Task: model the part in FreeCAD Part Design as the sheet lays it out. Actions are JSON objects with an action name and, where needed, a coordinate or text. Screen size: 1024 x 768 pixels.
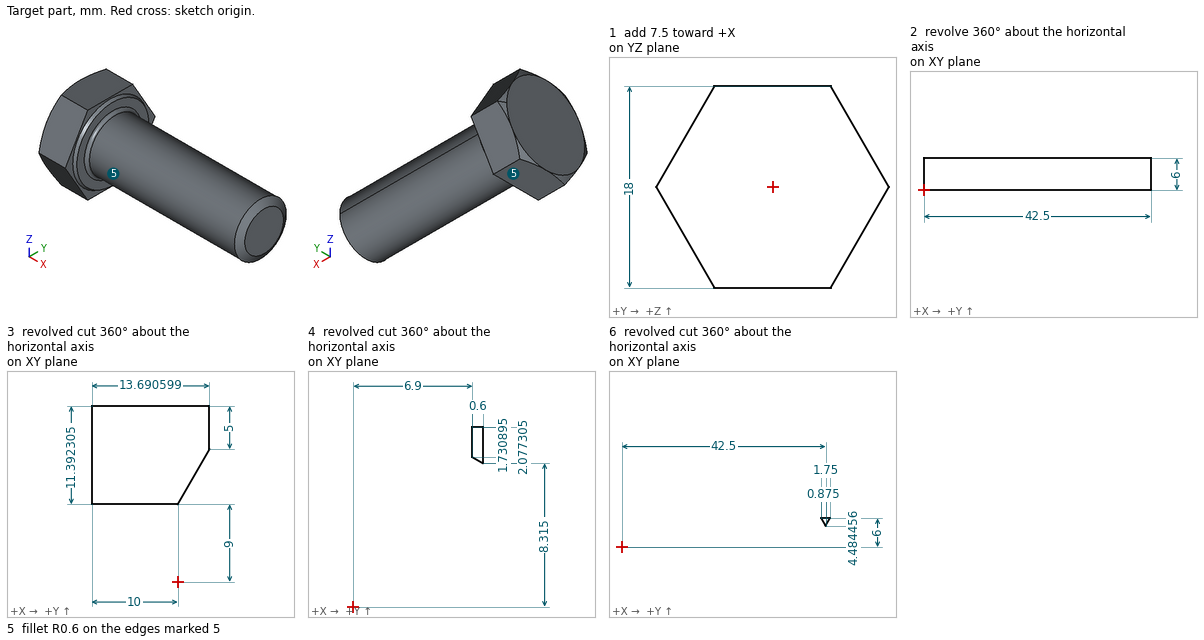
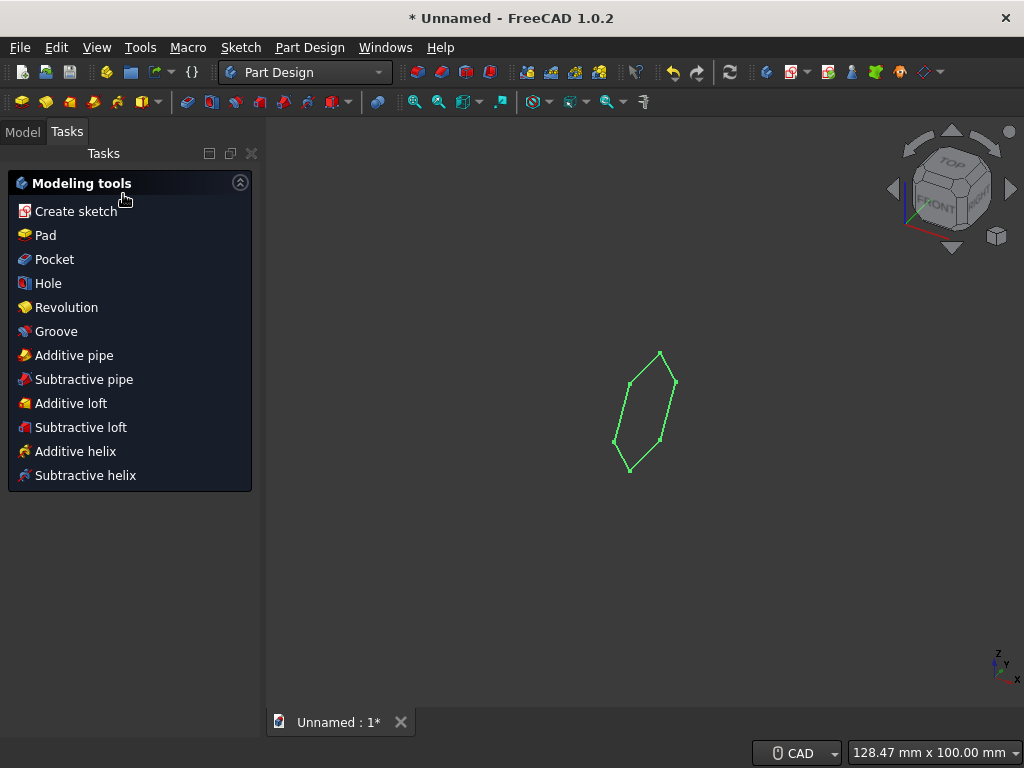
{"action": "left_click", "coordinate": [22, 102]}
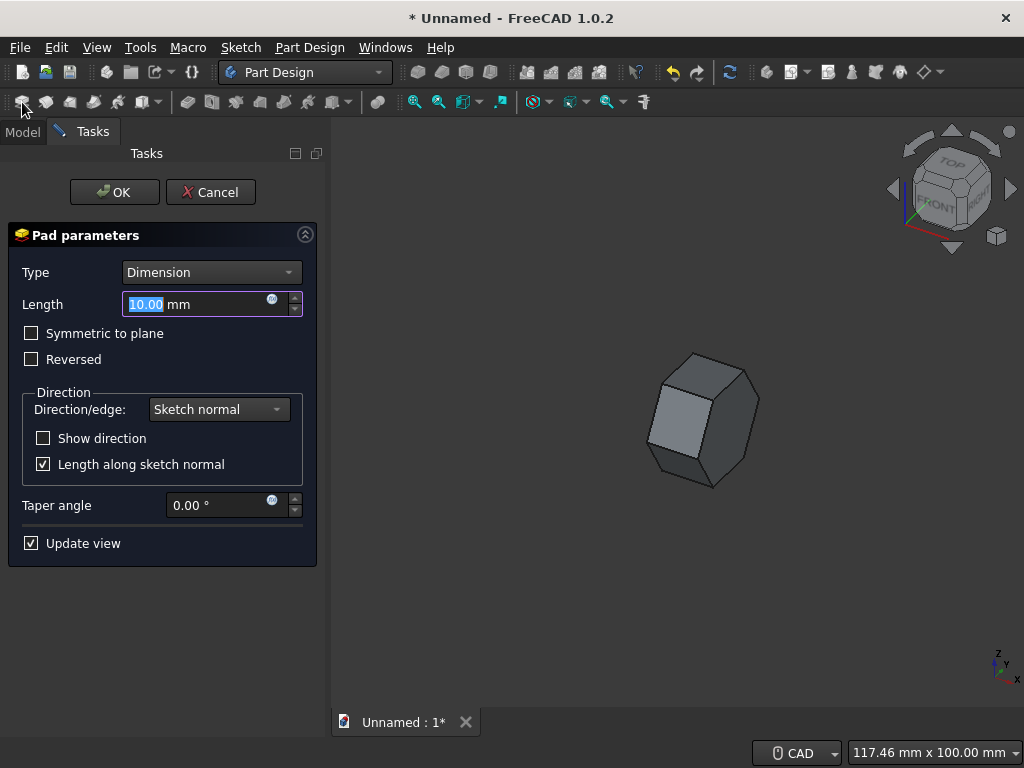
{"action": "type", "text": "7.5"}
{"action": "key", "text": "Tab"}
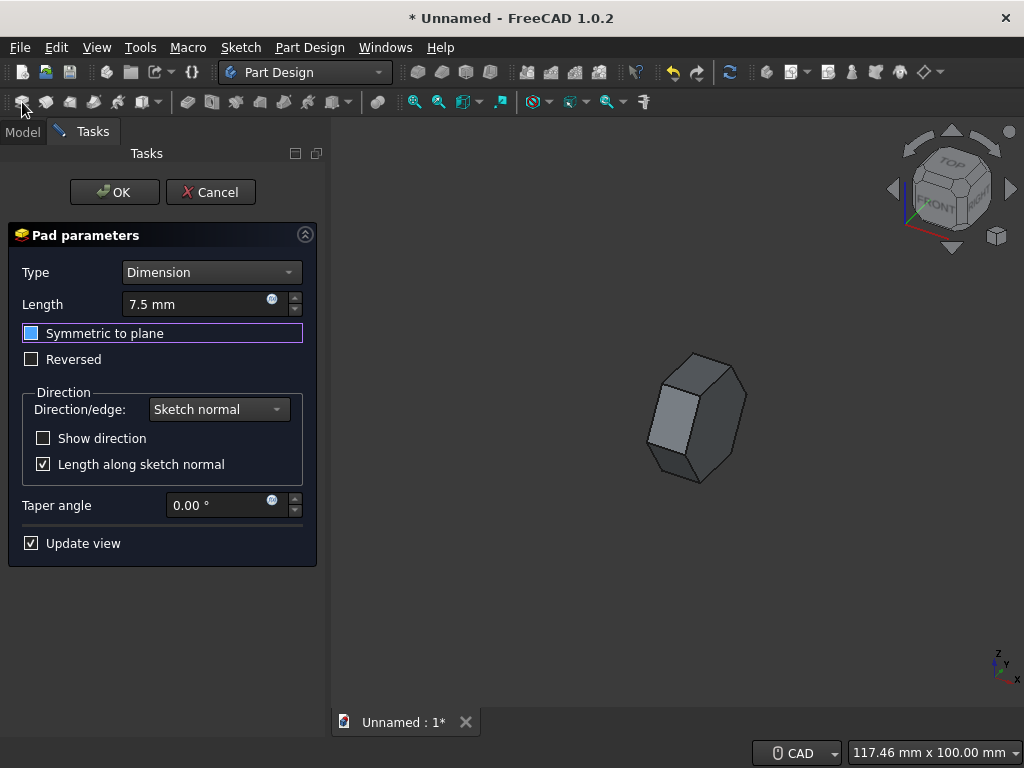
{"action": "left_click", "coordinate": [115, 192]}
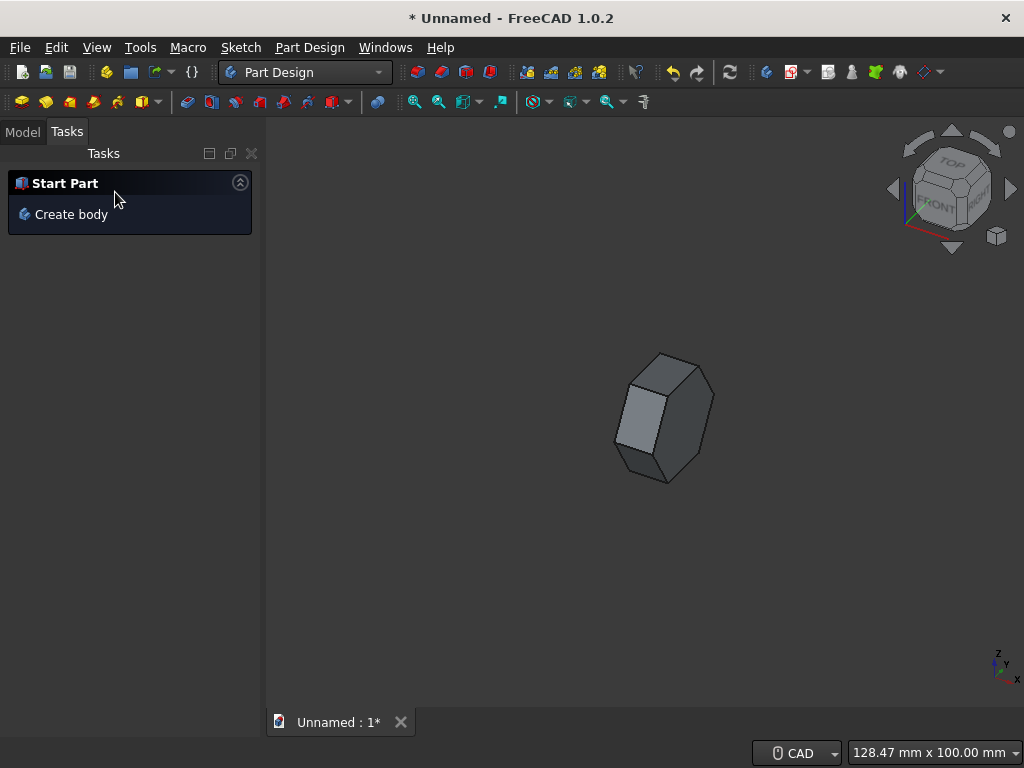
{"action": "left_click", "coordinate": [416, 102]}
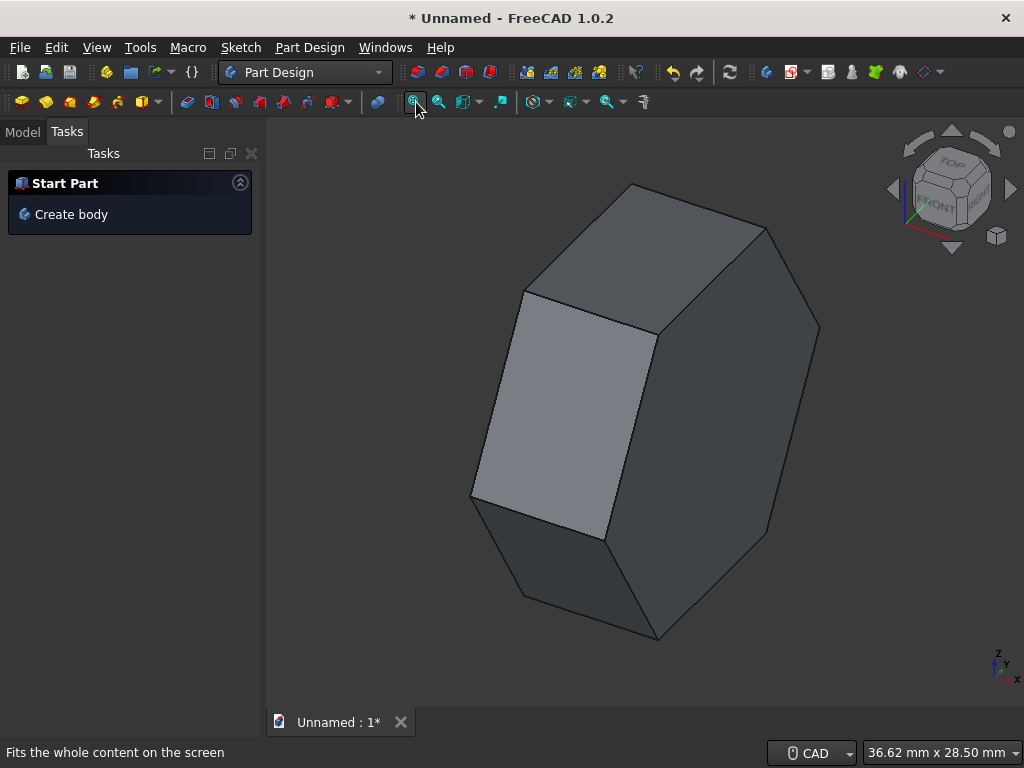
{"action": "left_click", "coordinate": [792, 72]}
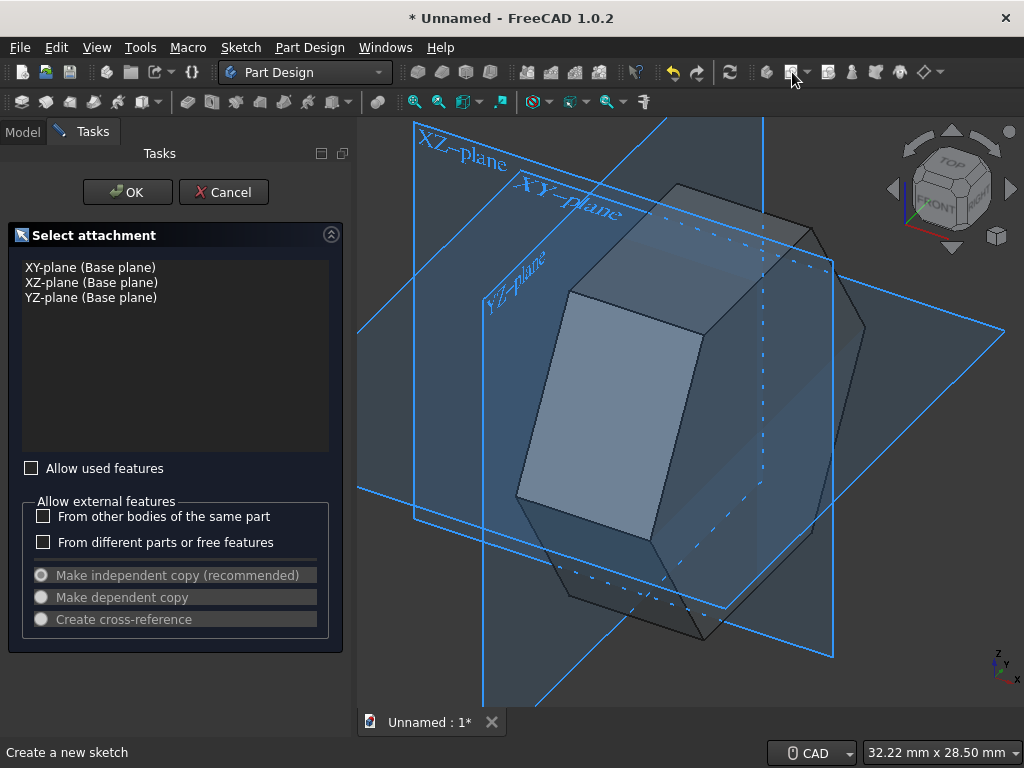
{"action": "left_click", "coordinate": [82, 268]}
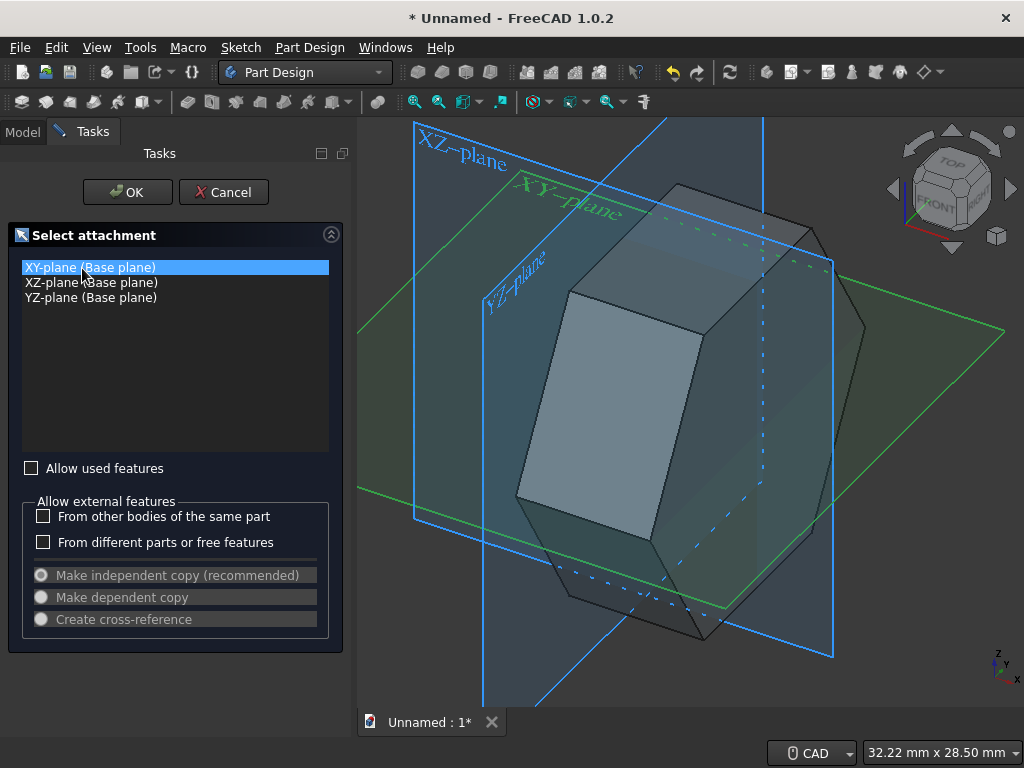
{"action": "left_click", "coordinate": [128, 192]}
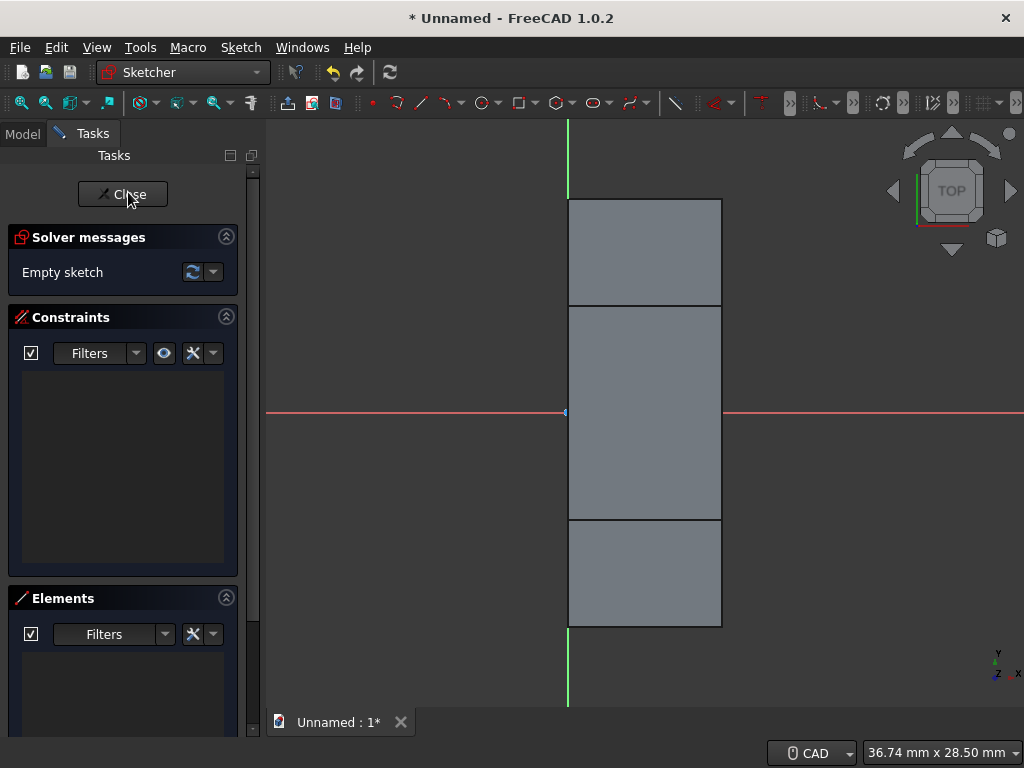
{"action": "left_click", "coordinate": [336, 104]}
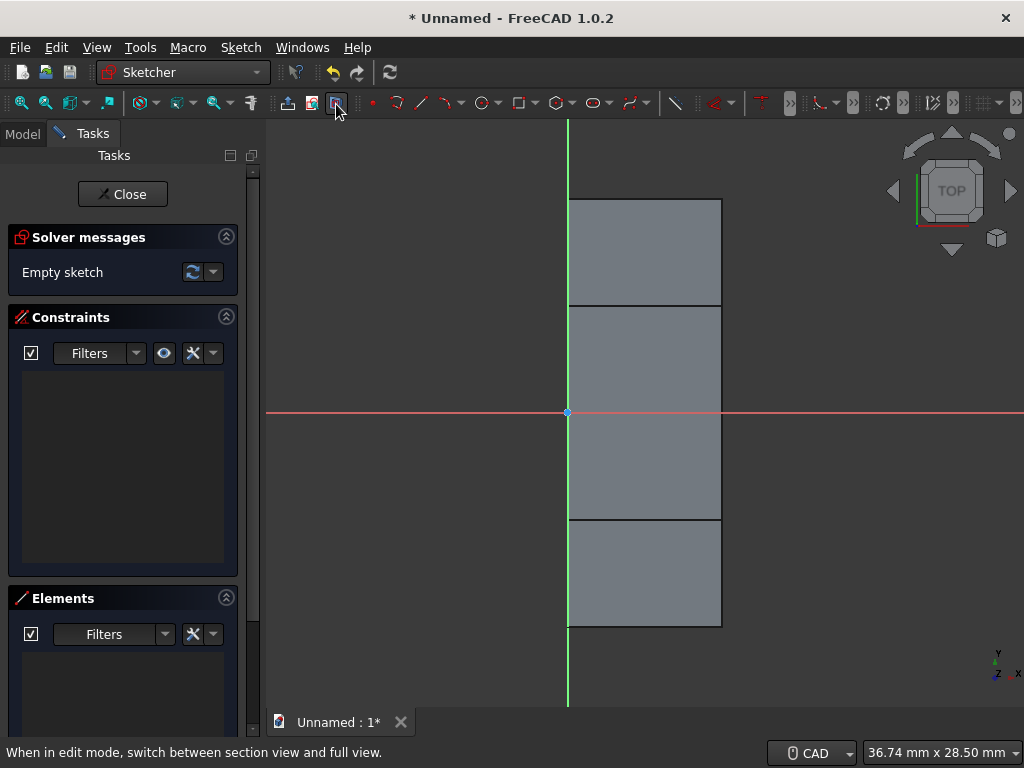
{"action": "scroll", "coordinate": [294, 464], "scroll_direction": "down", "scroll_amount": 4}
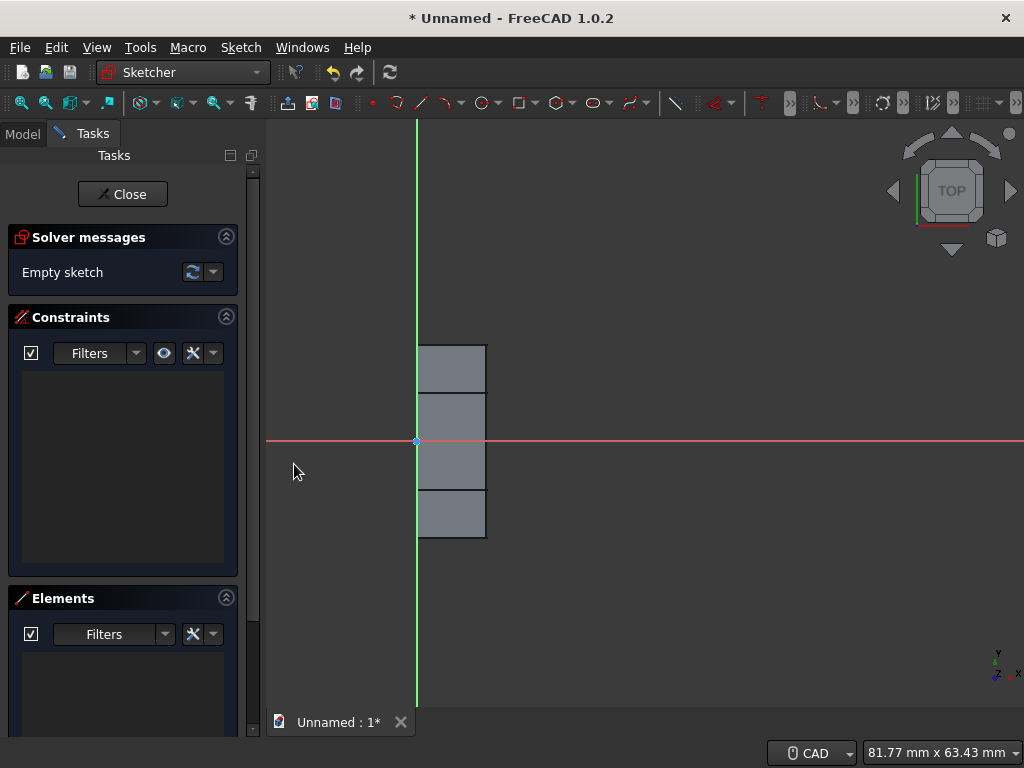
{"action": "left_click", "coordinate": [520, 104]}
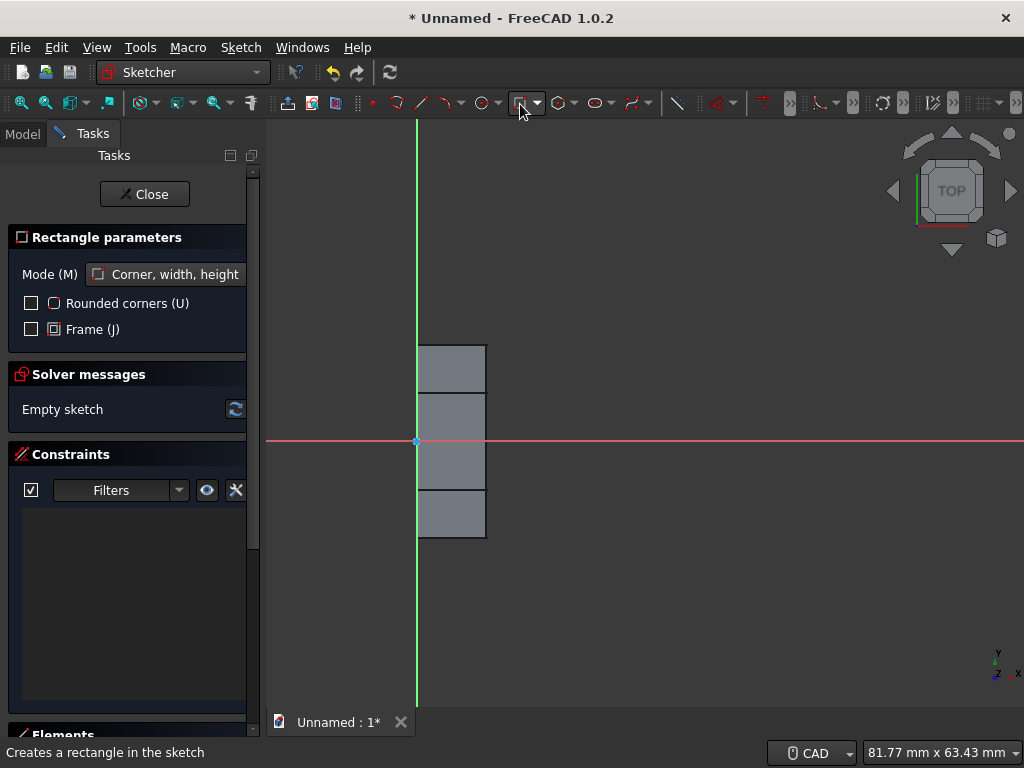
{"action": "left_click", "coordinate": [417, 441]}
{"action": "mouse_move", "coordinate": [811, 386]}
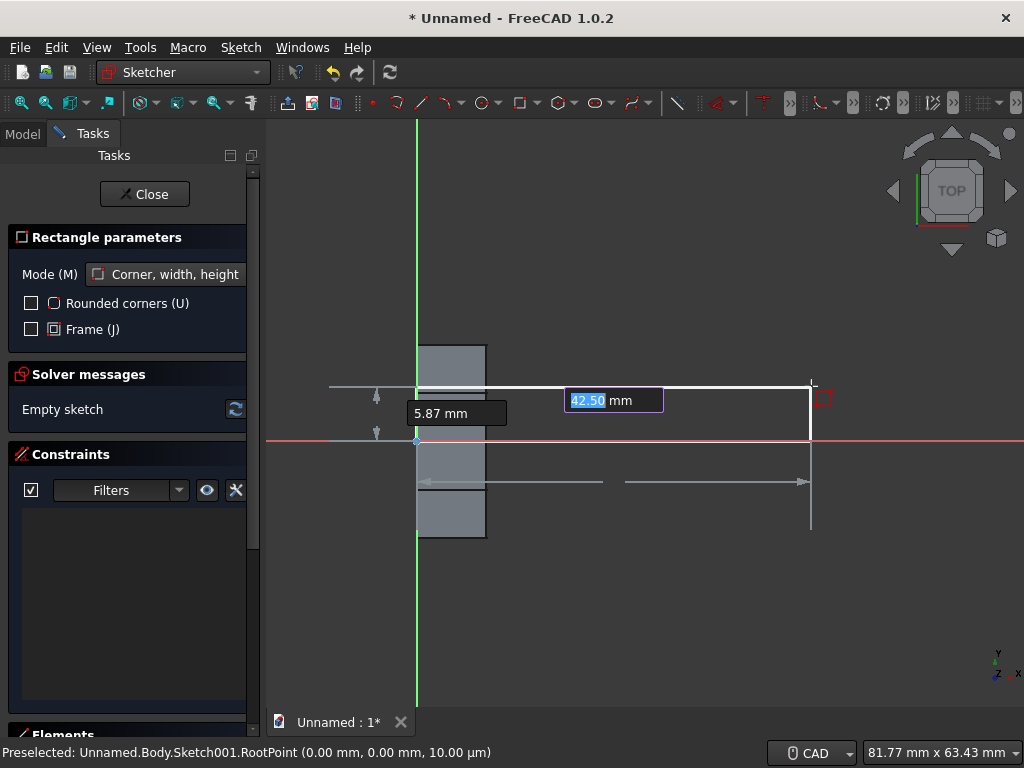
{"action": "type", "text": "42.5"}
{"action": "key", "text": "Tab"}
{"action": "type", "text": "6"}
{"action": "key", "text": "Return"}
{"action": "key", "text": "Escape"}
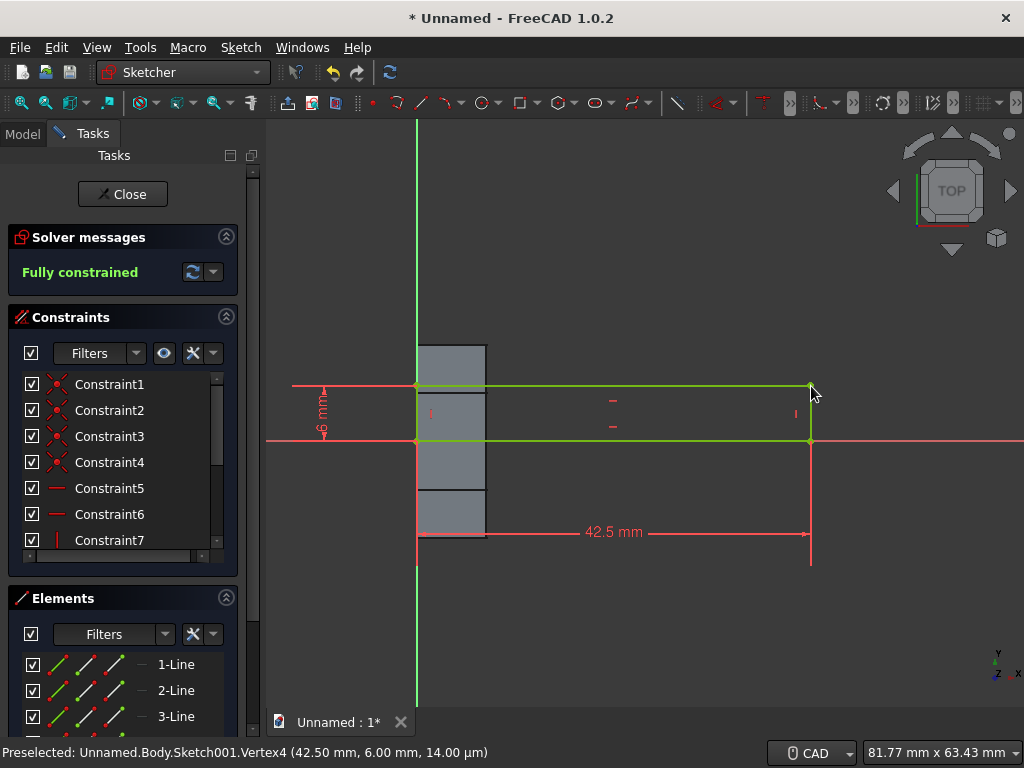
{"action": "left_click", "coordinate": [123, 194]}